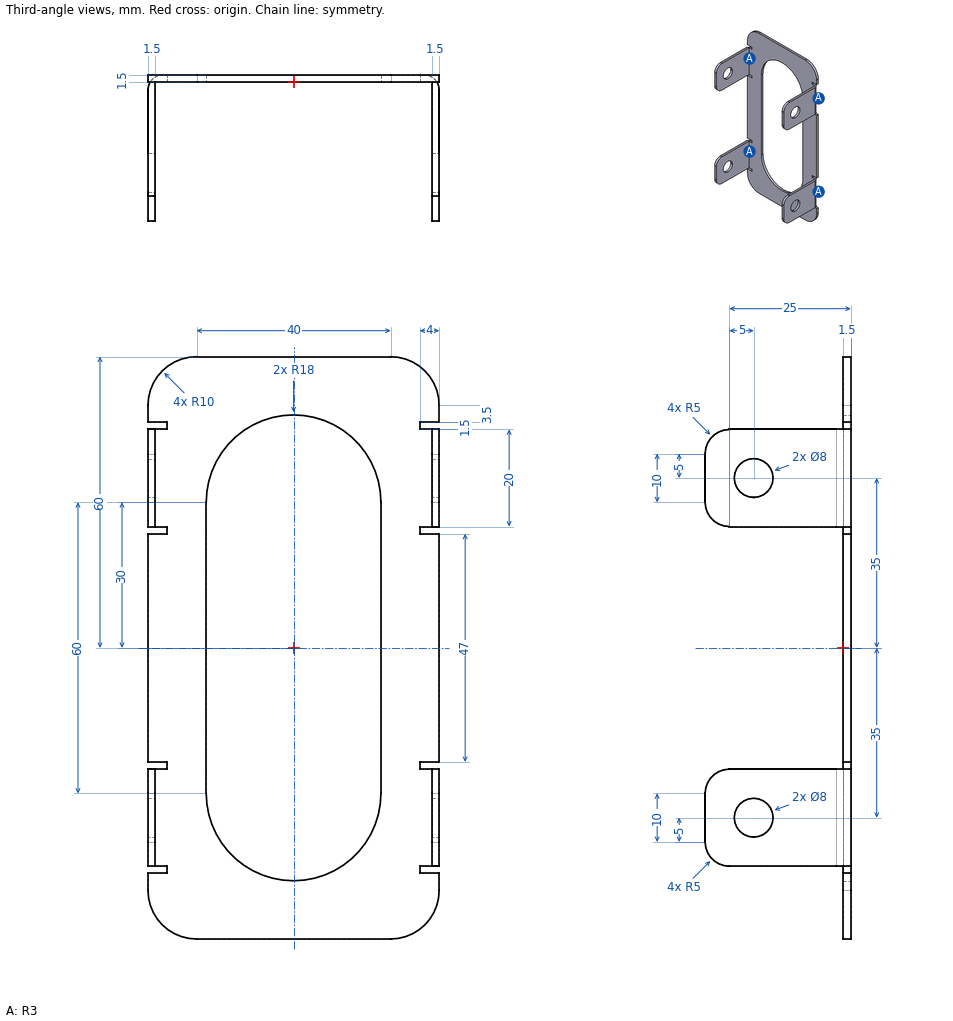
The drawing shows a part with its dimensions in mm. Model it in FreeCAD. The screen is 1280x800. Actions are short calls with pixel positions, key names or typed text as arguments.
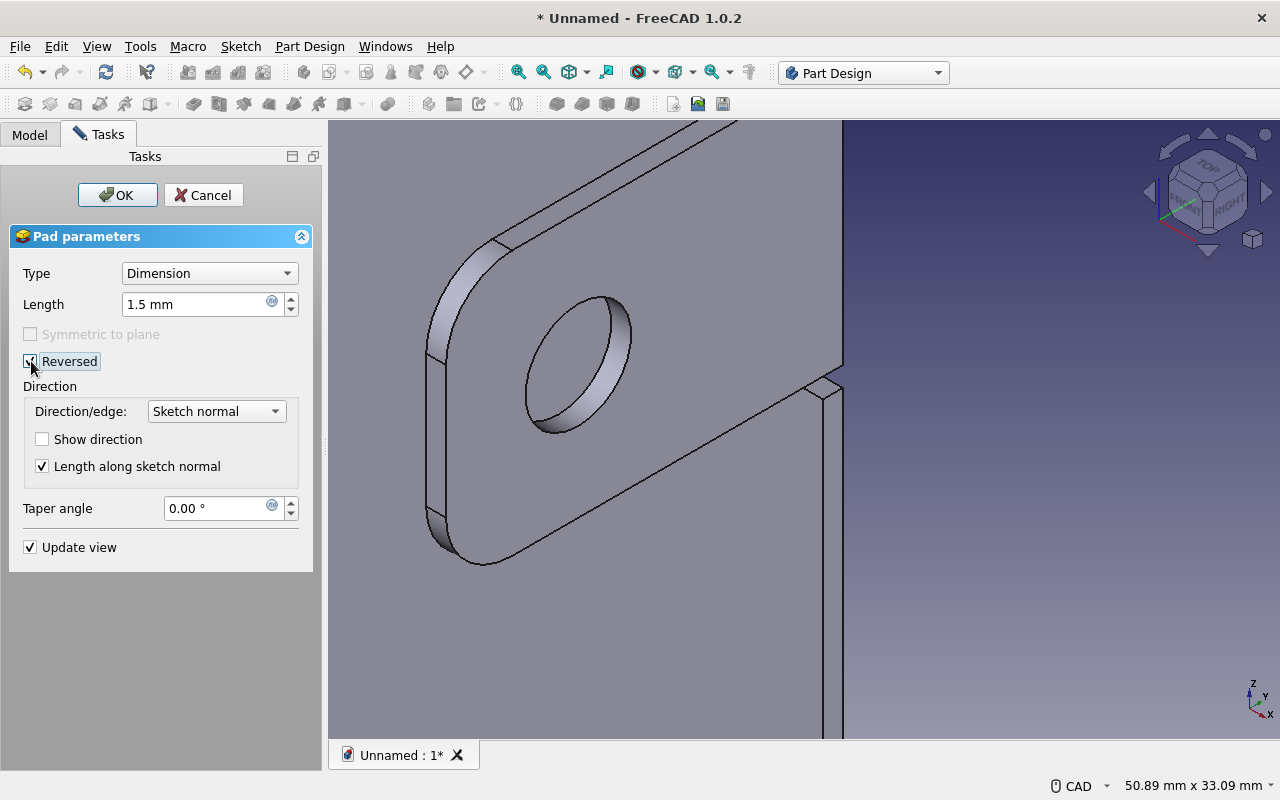
click(118, 195)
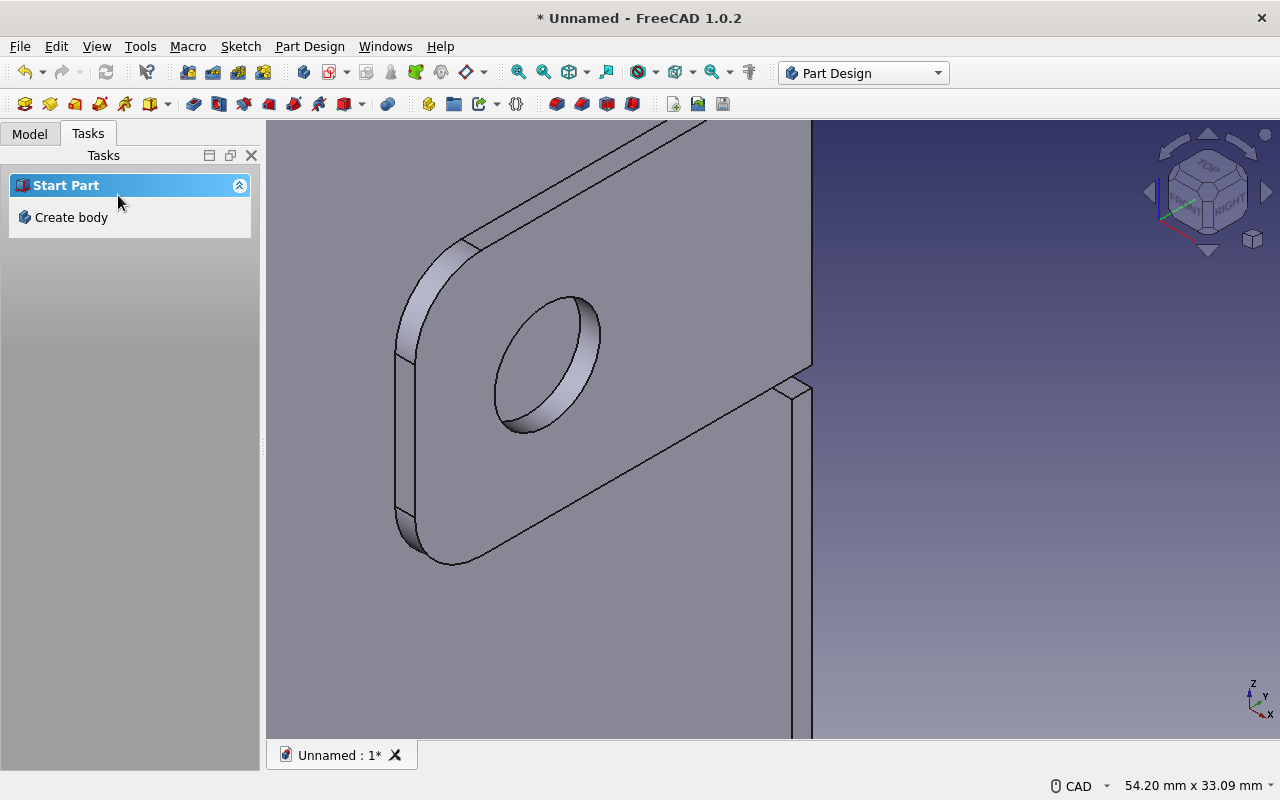
click(519, 72)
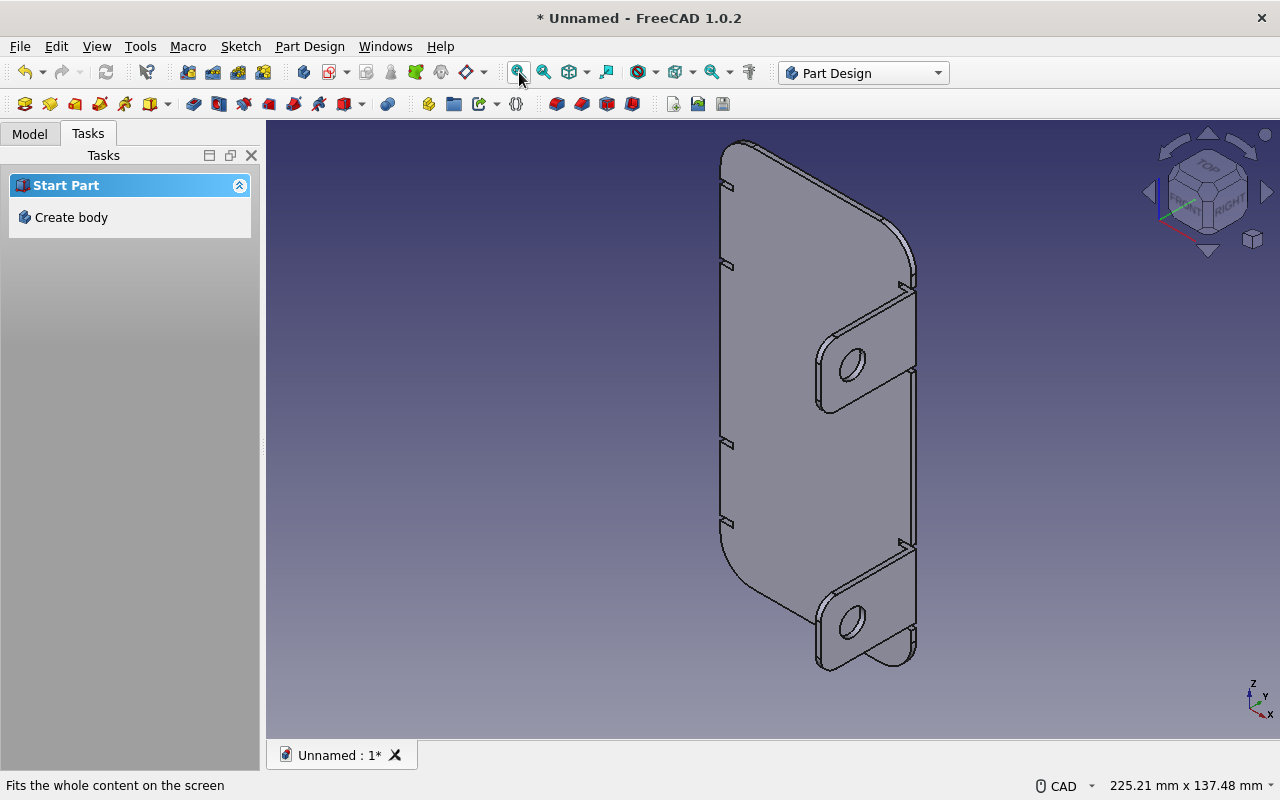
click(30, 134)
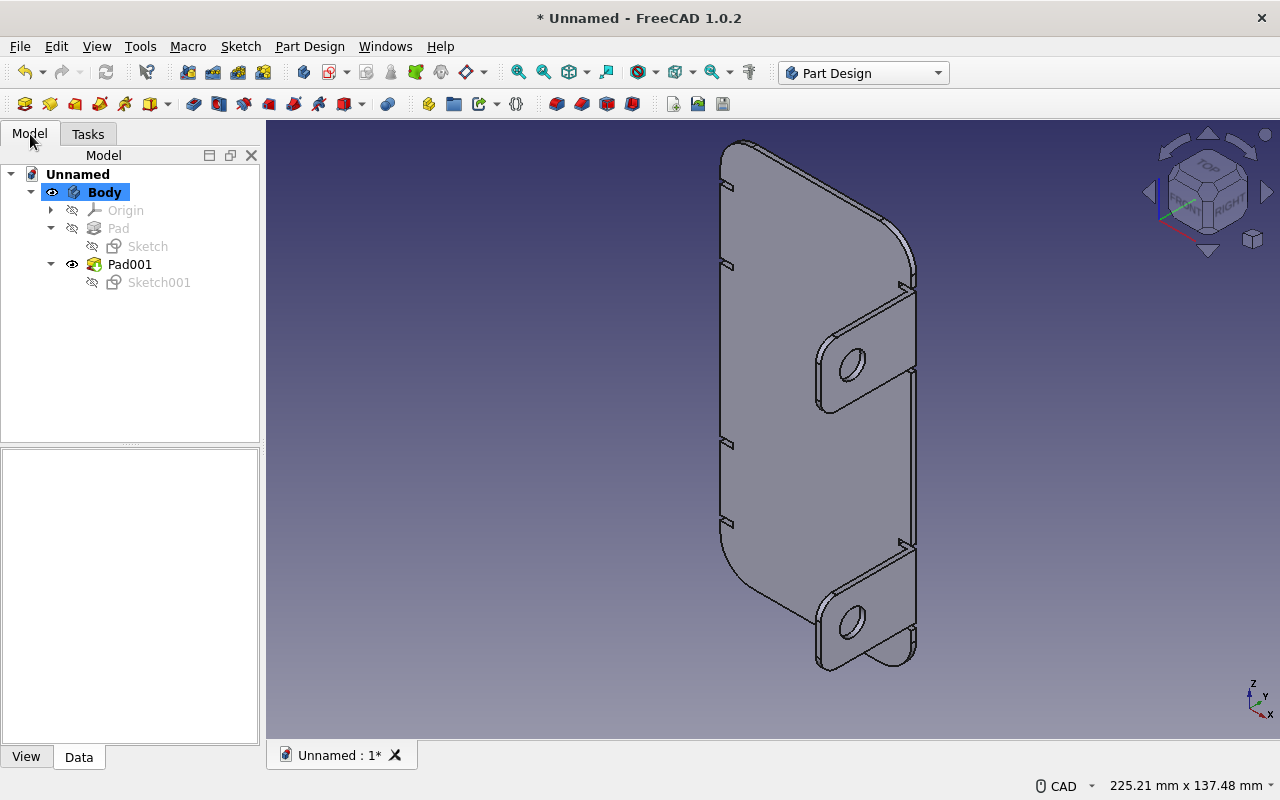
click(51, 210)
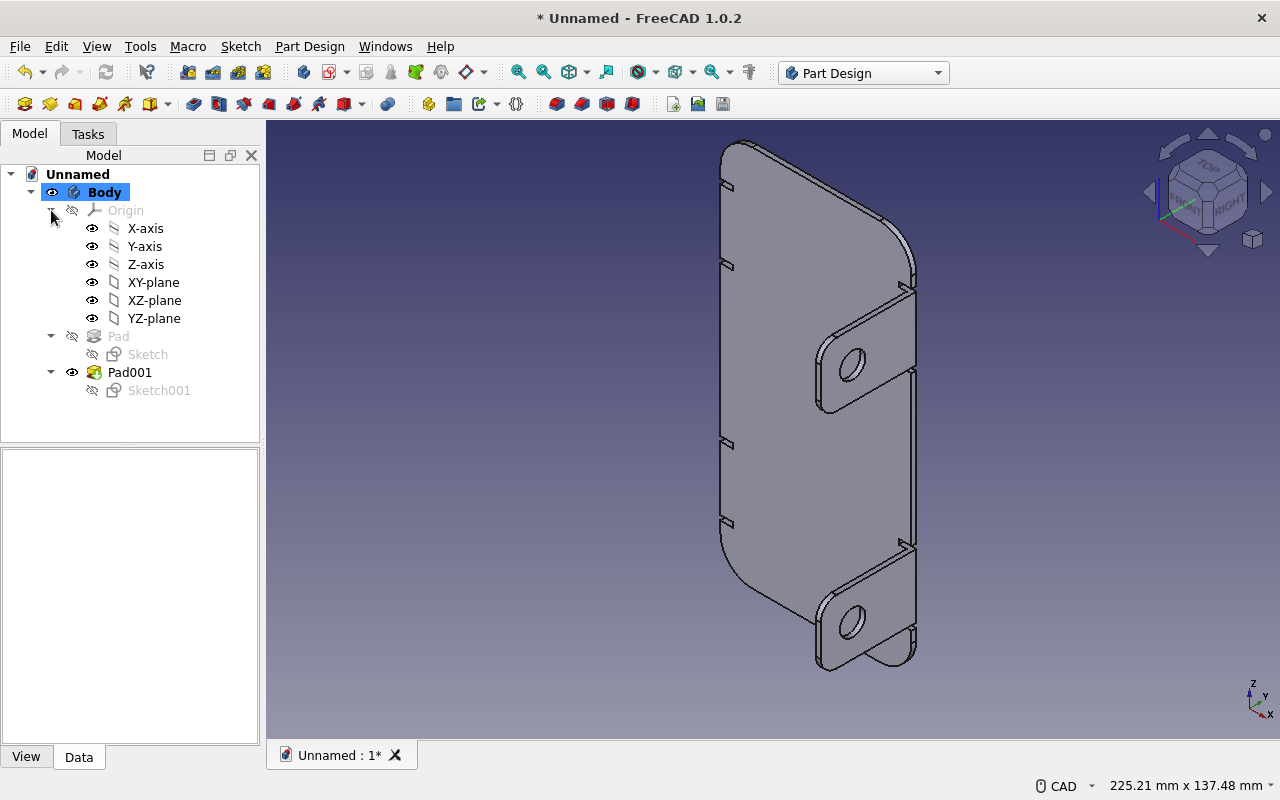
click(137, 318)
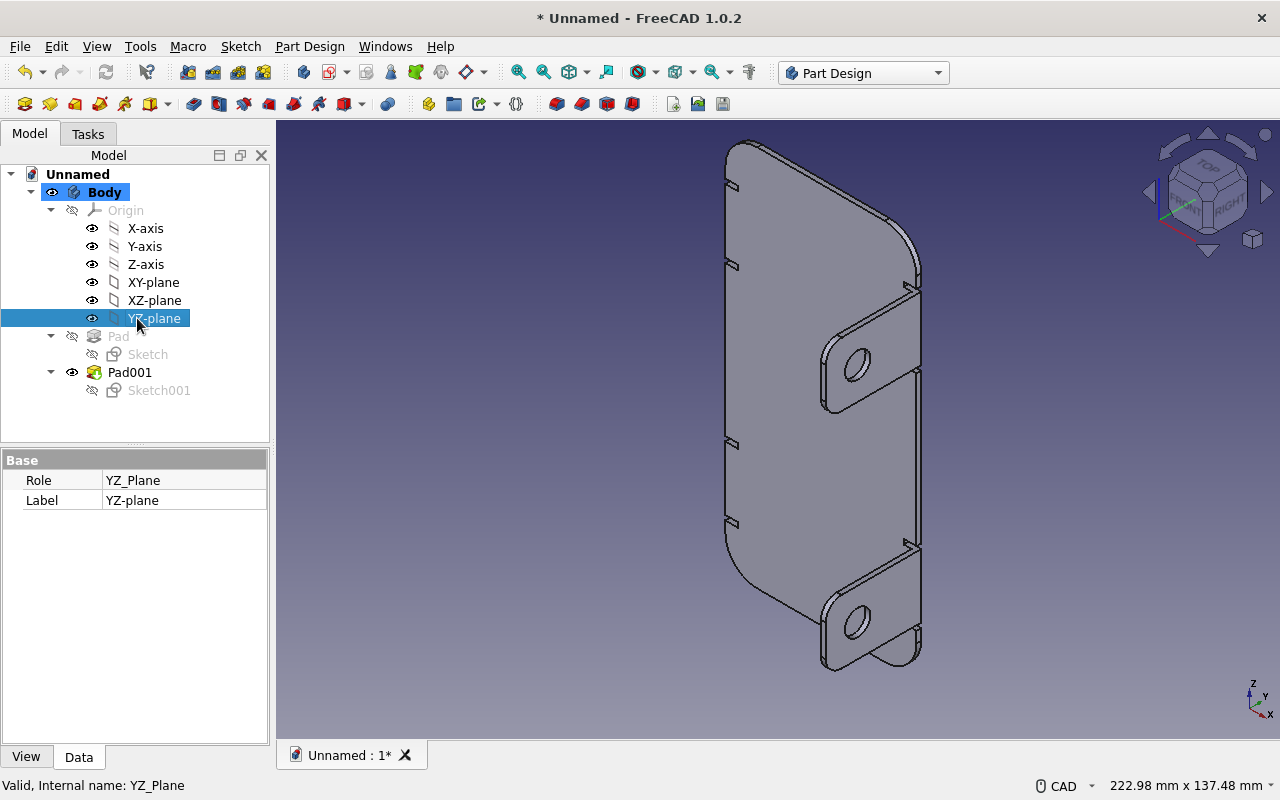
click(466, 72)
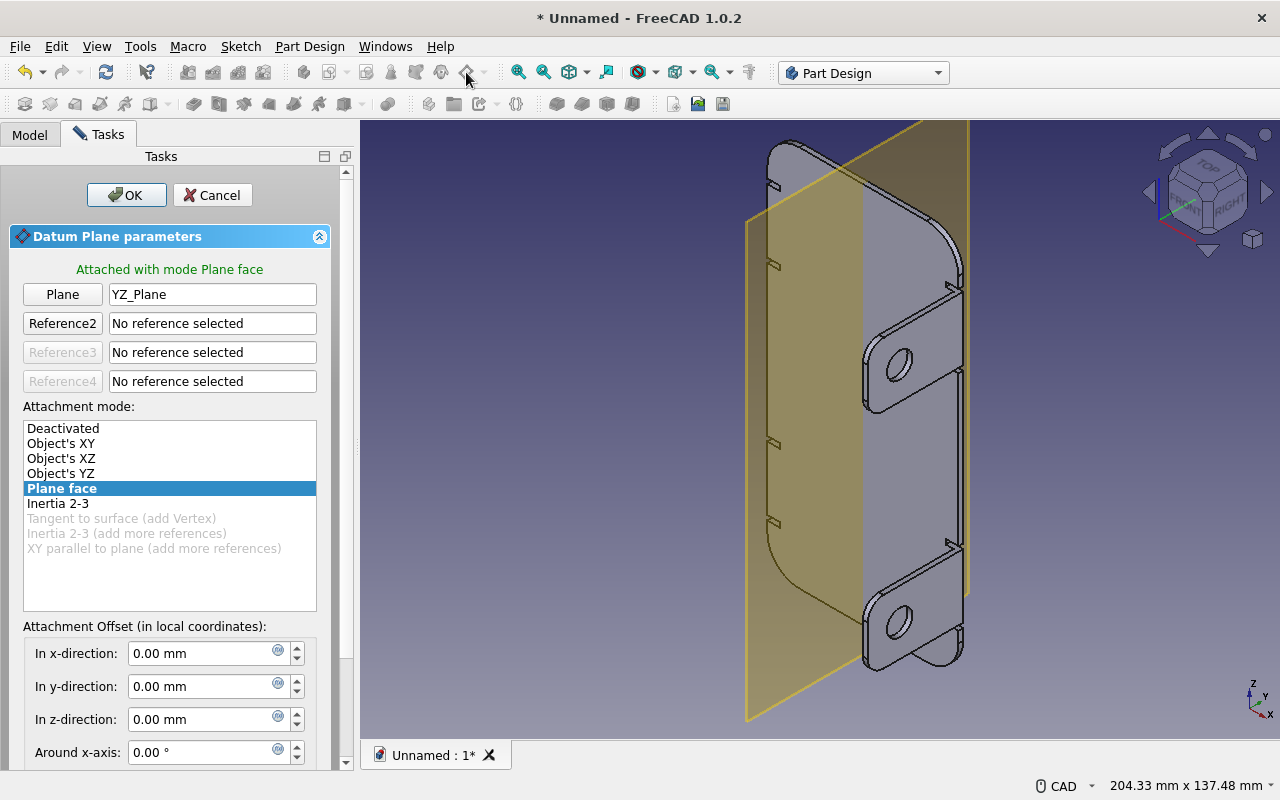
triple_click(210, 720)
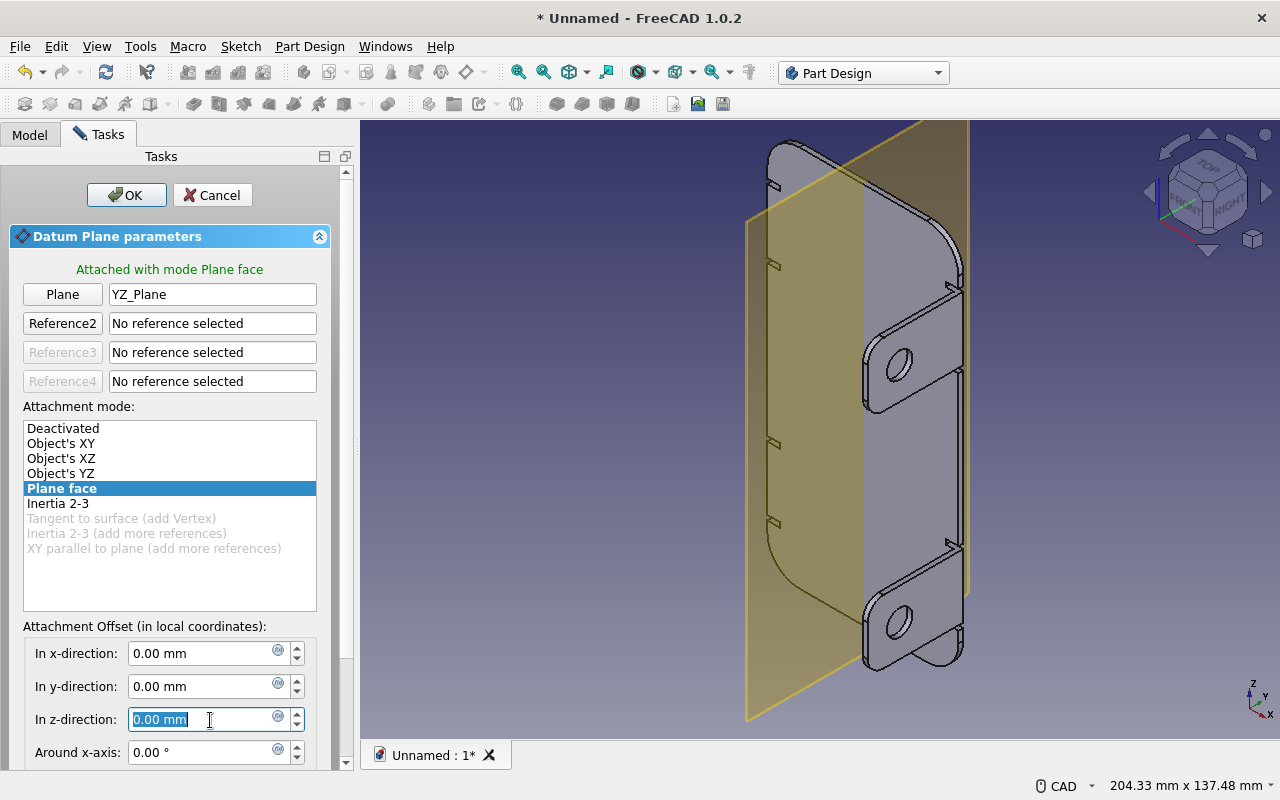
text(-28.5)
key(Tab)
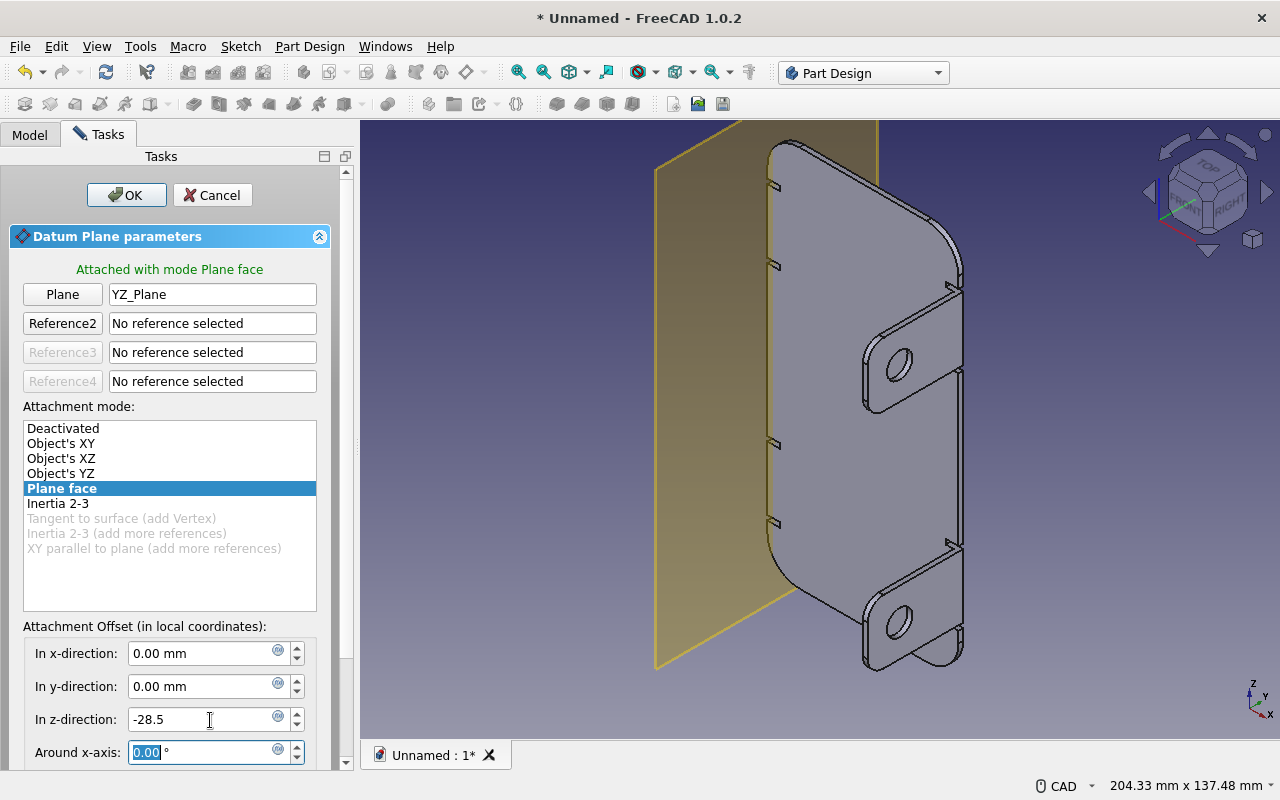
click(127, 195)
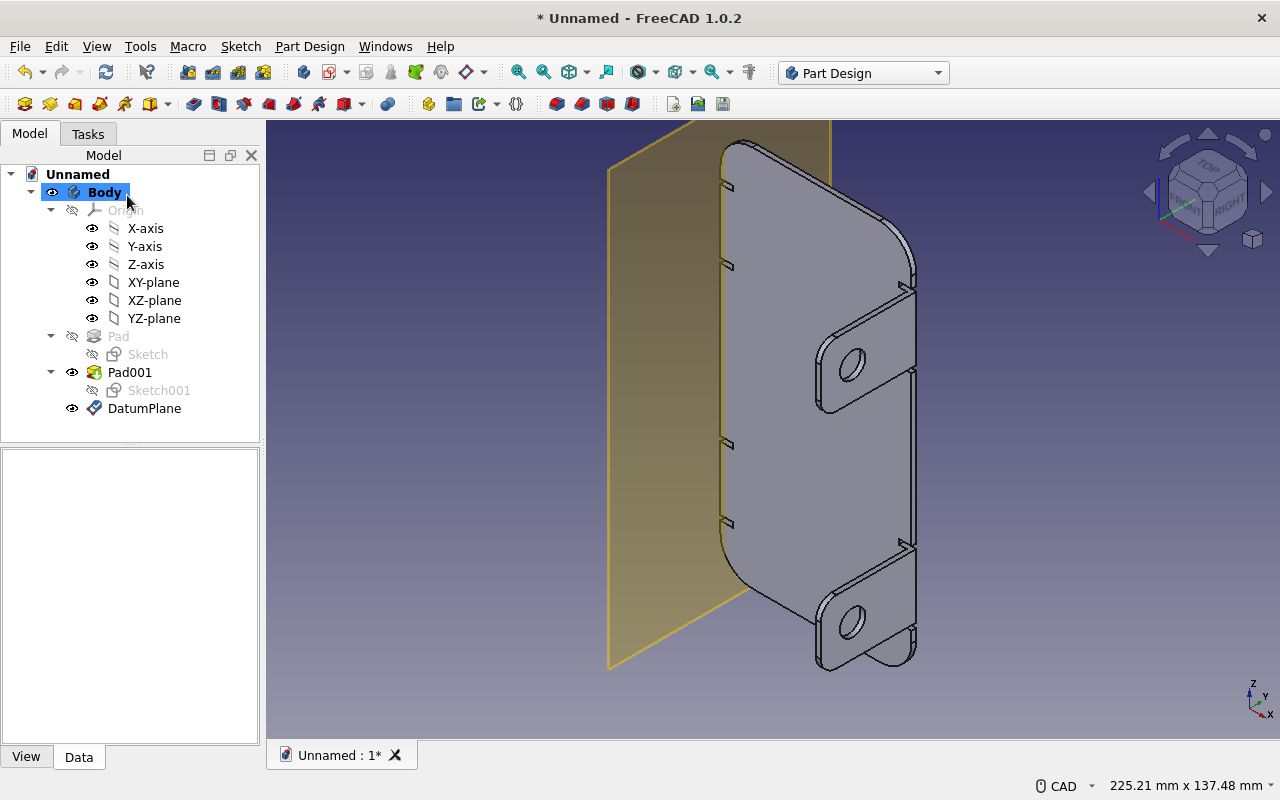
click(117, 408)